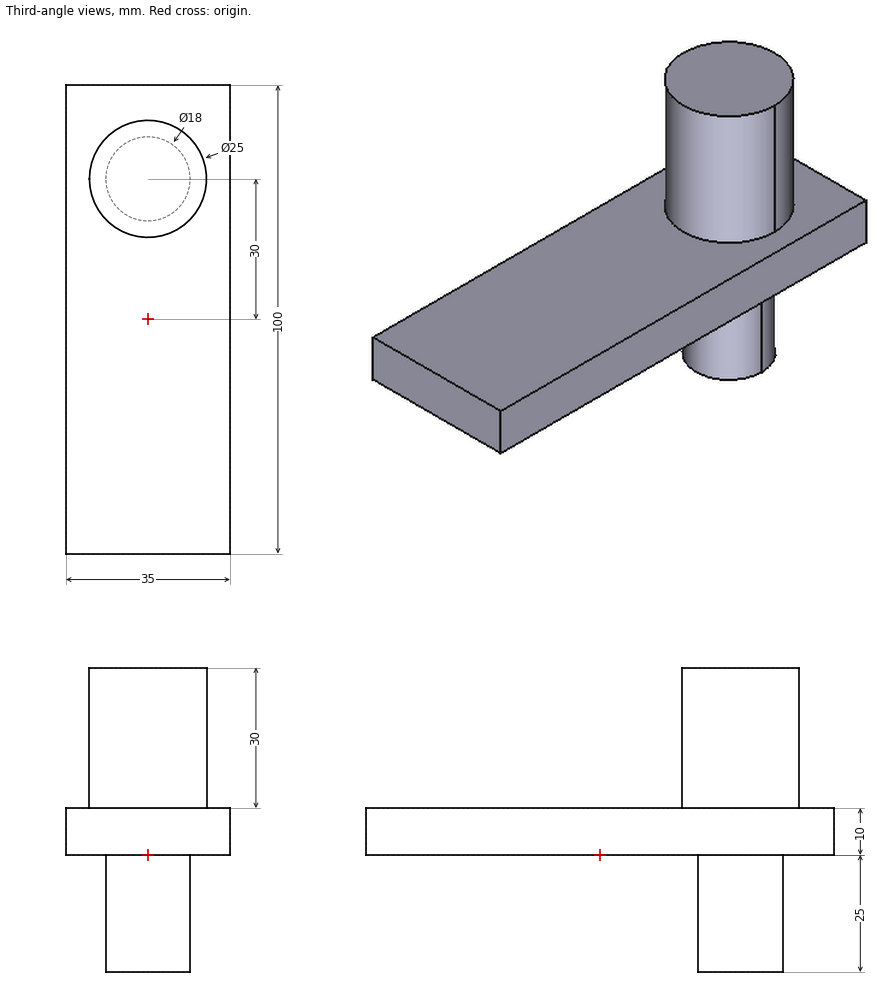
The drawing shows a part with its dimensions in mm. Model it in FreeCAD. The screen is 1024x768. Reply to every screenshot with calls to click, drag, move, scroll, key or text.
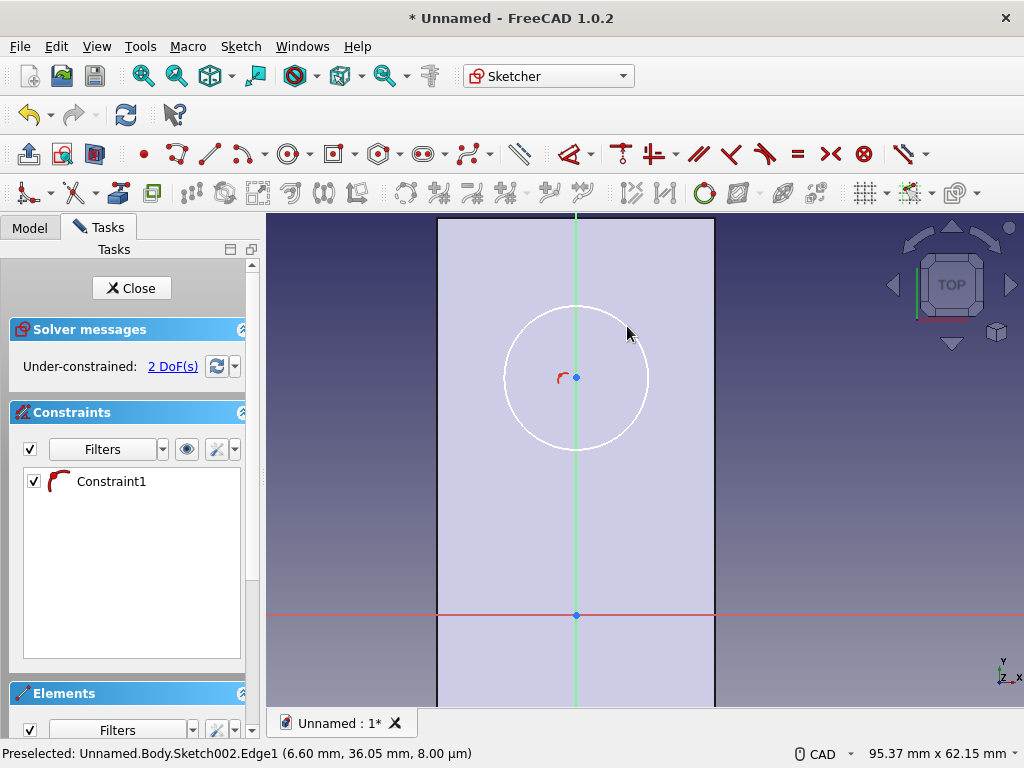
click(568, 154)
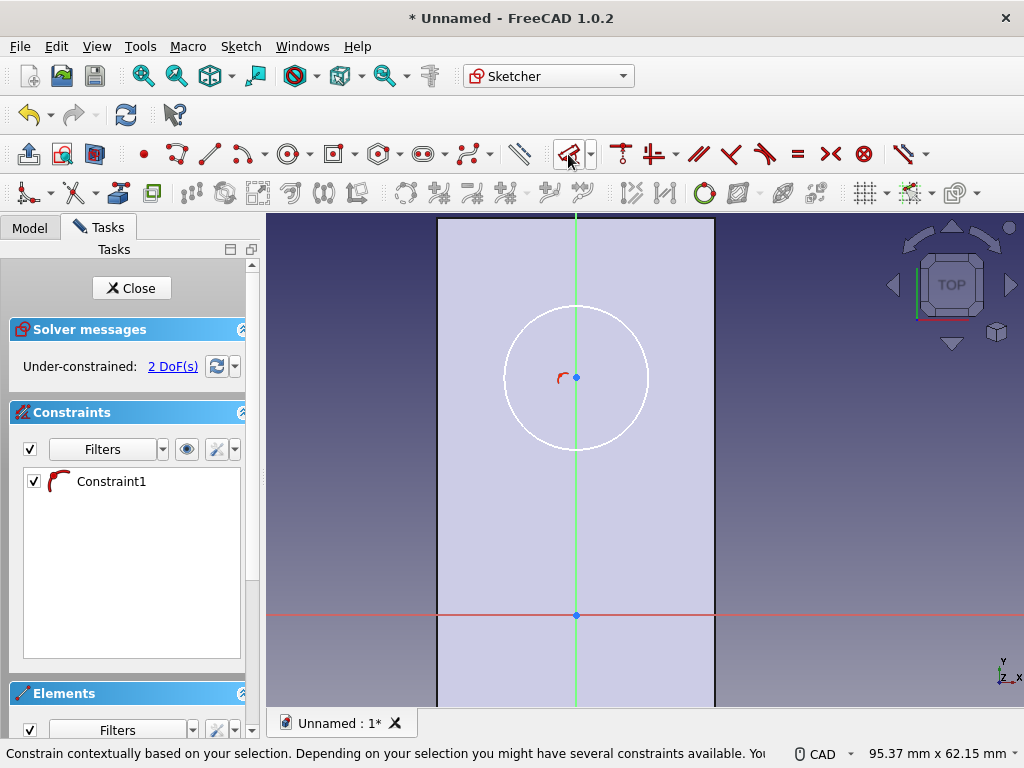
click(627, 327)
click(650, 304)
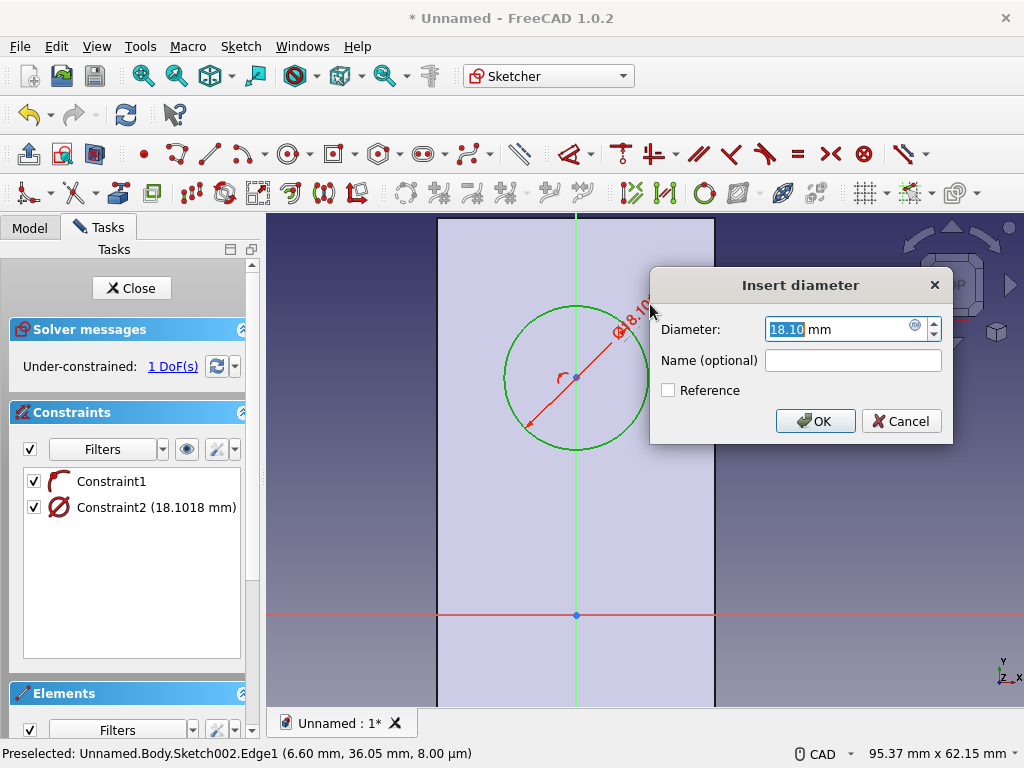
text(18)
key(Return)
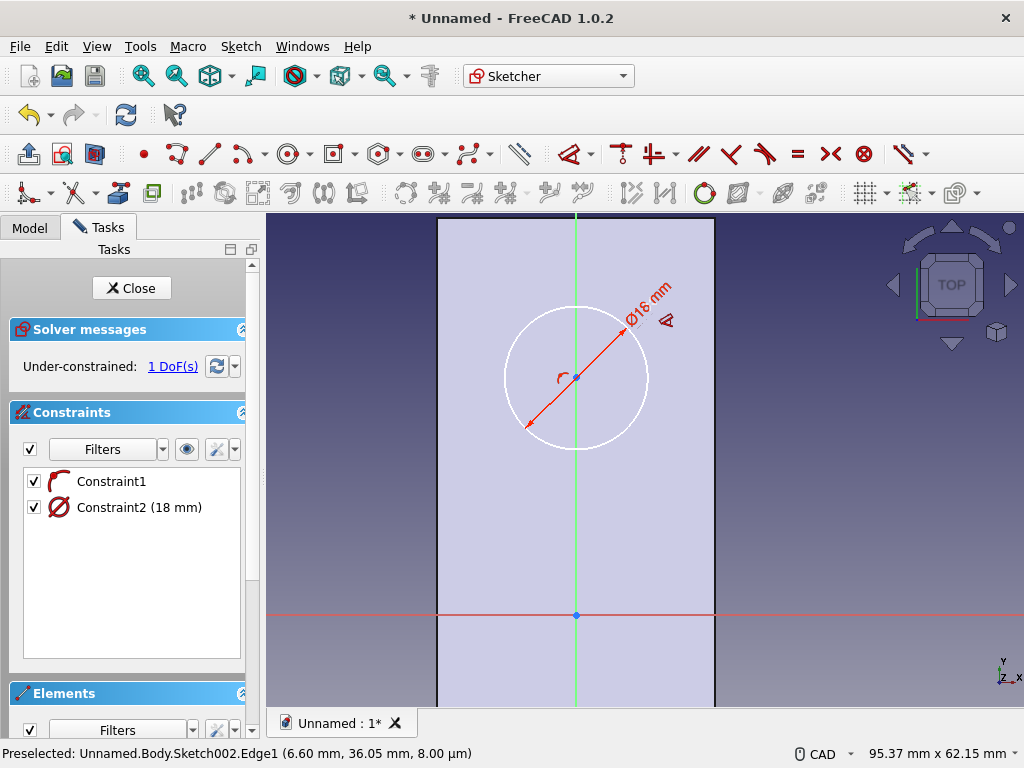
click(576, 378)
click(610, 497)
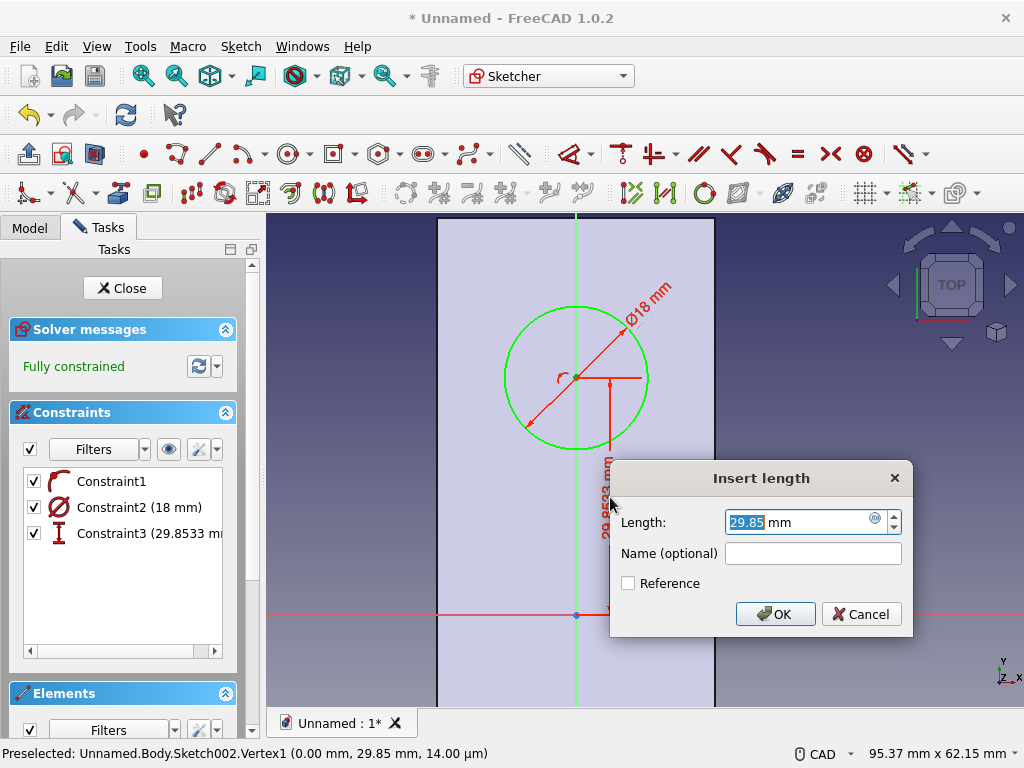
text(30)
key(Return)
key(Escape)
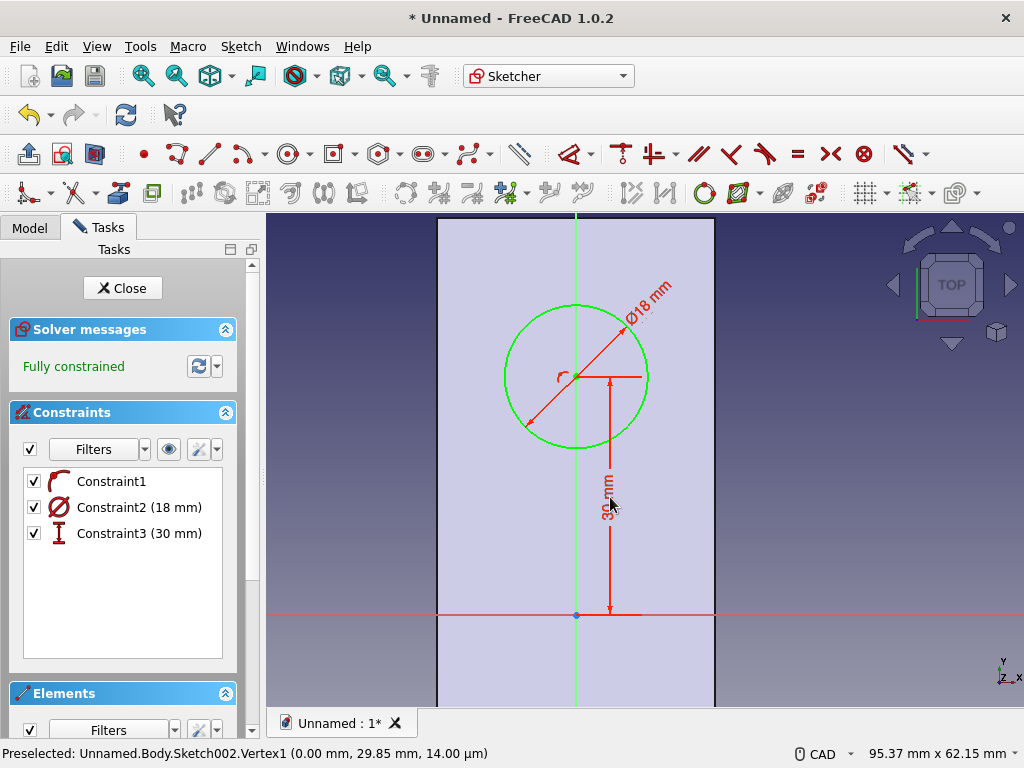
click(123, 288)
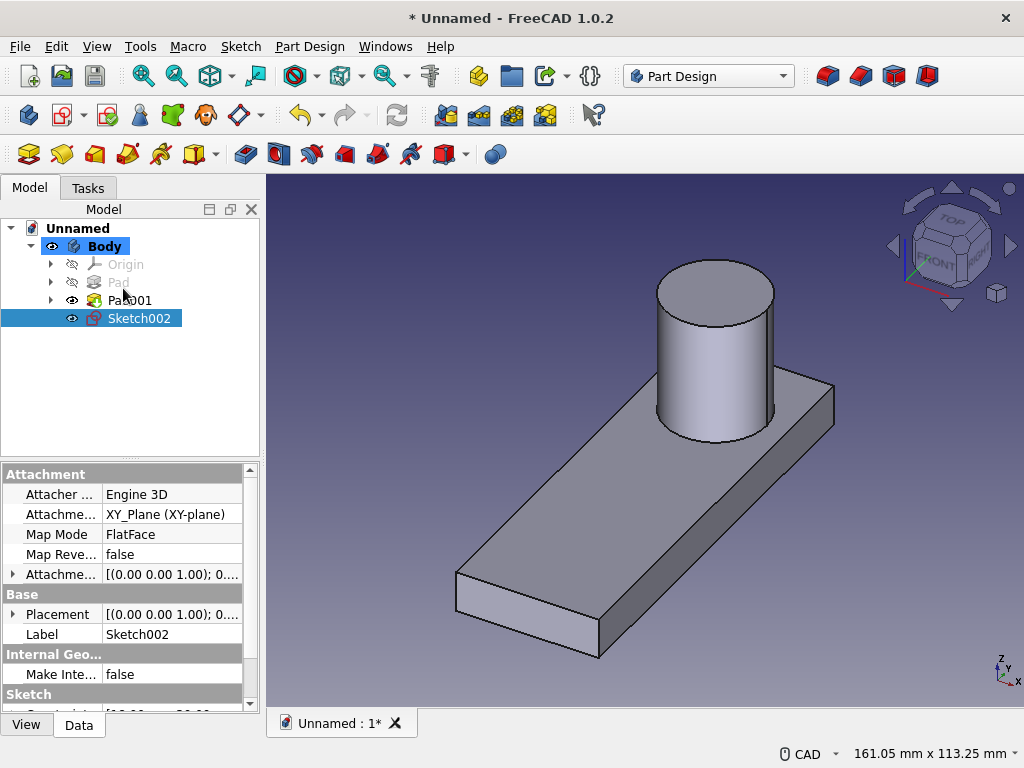
click(29, 154)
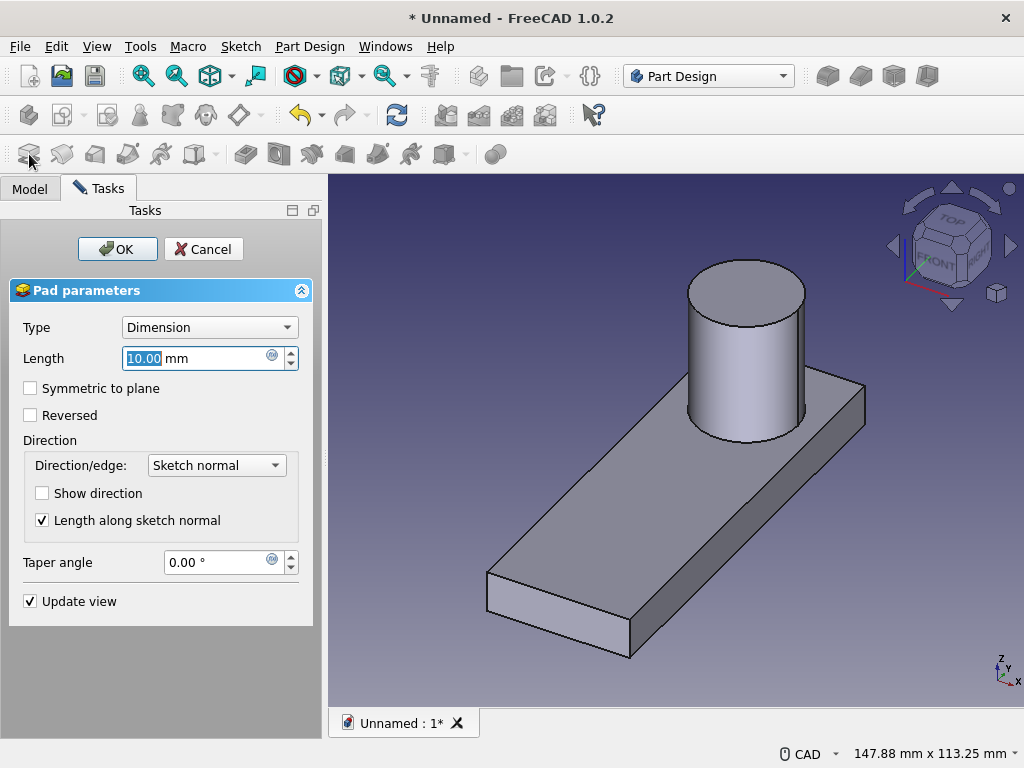
text(25)
key(Tab)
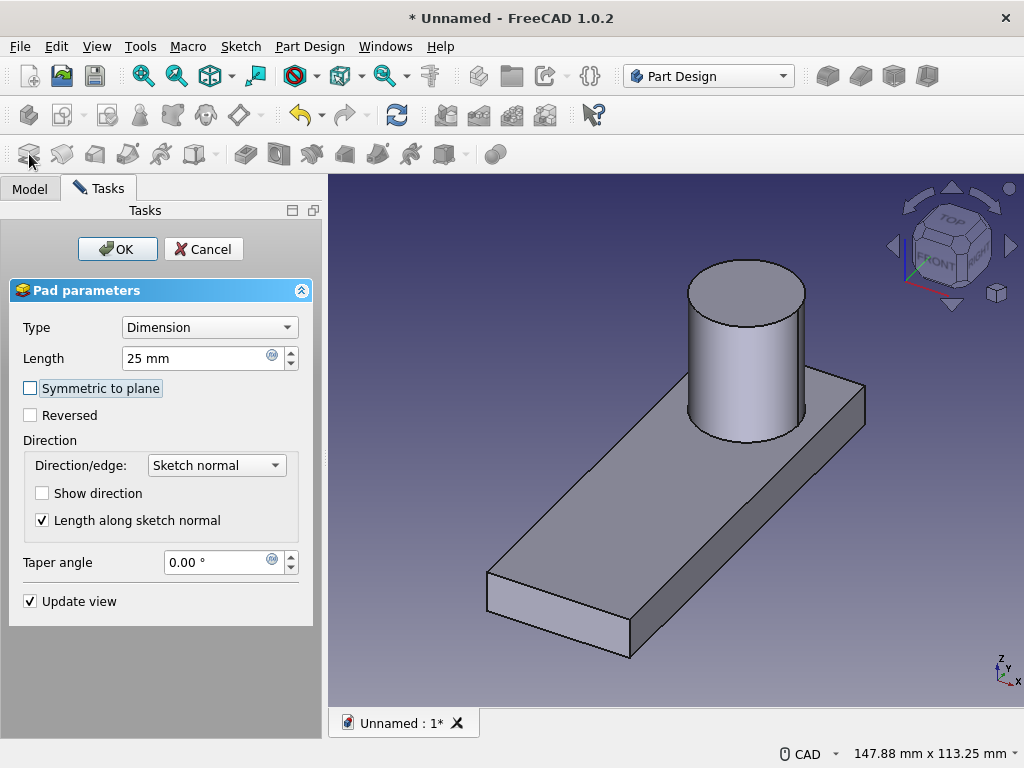
click(31, 415)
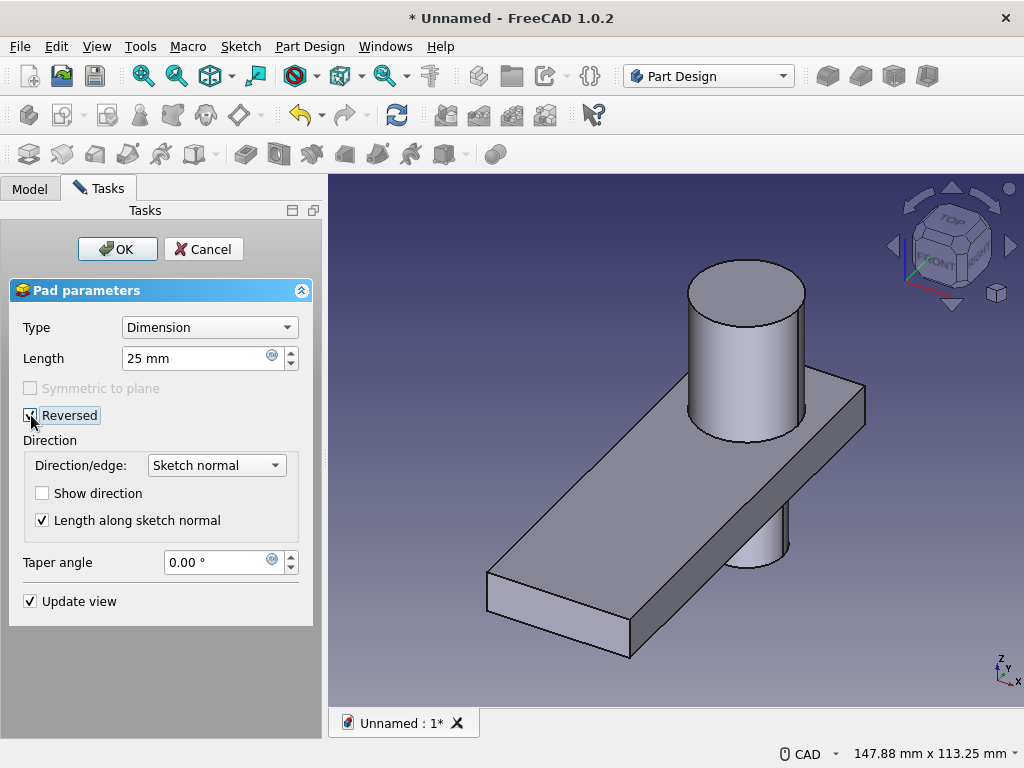
click(118, 249)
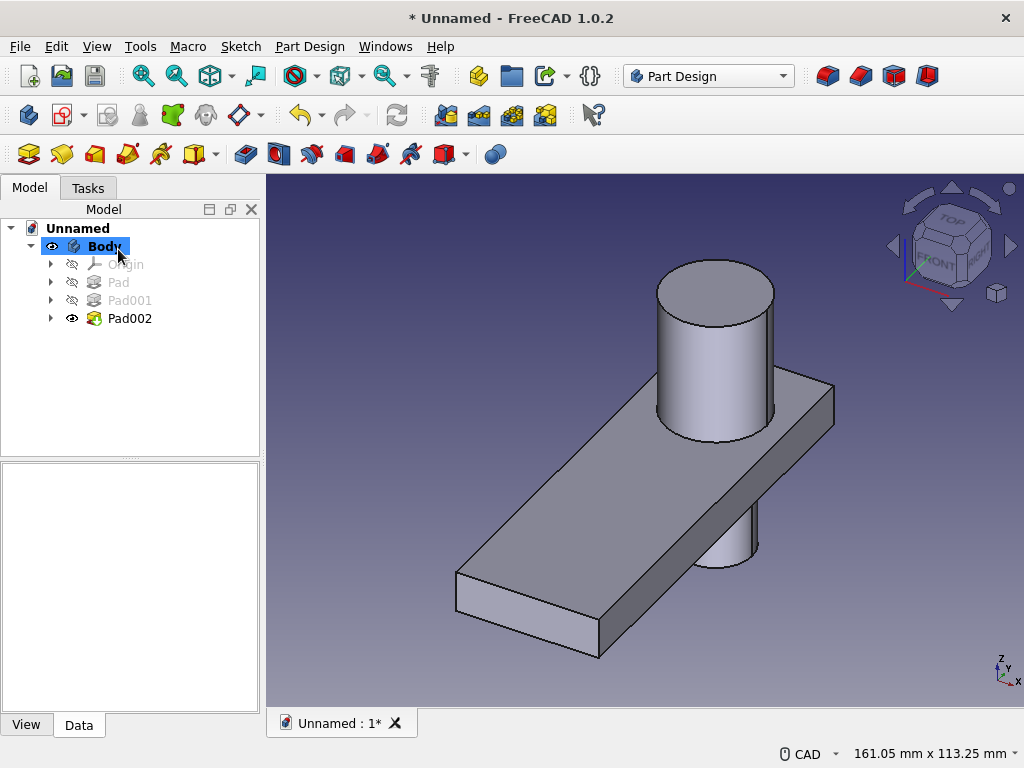
key(0)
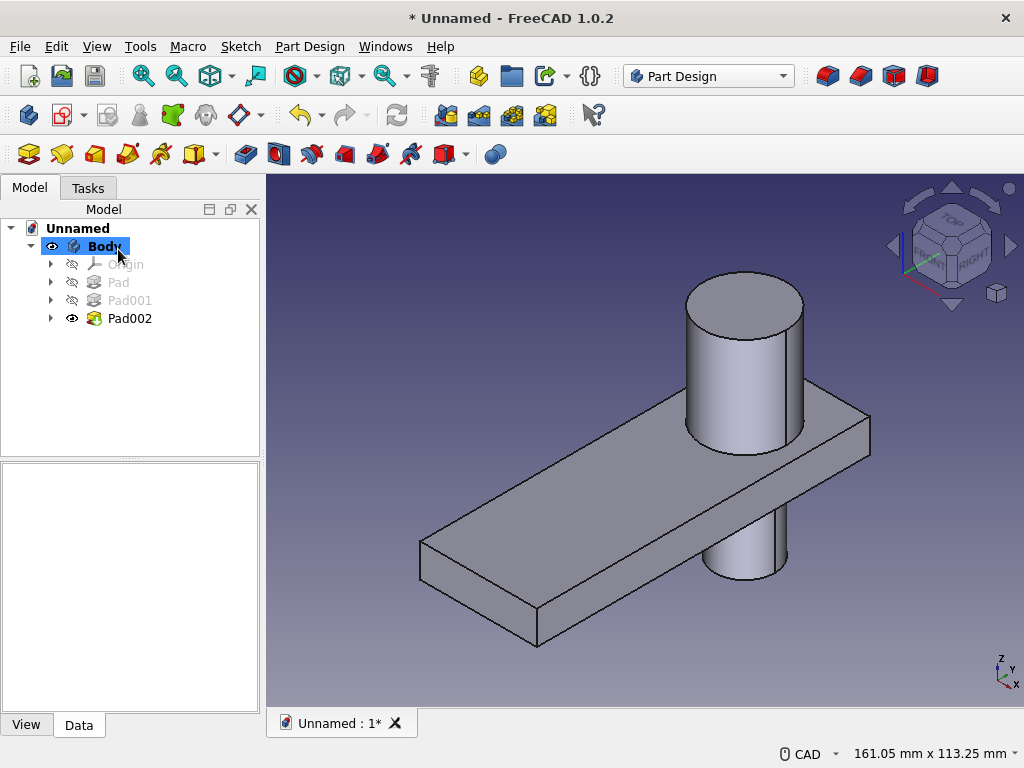
click(144, 76)